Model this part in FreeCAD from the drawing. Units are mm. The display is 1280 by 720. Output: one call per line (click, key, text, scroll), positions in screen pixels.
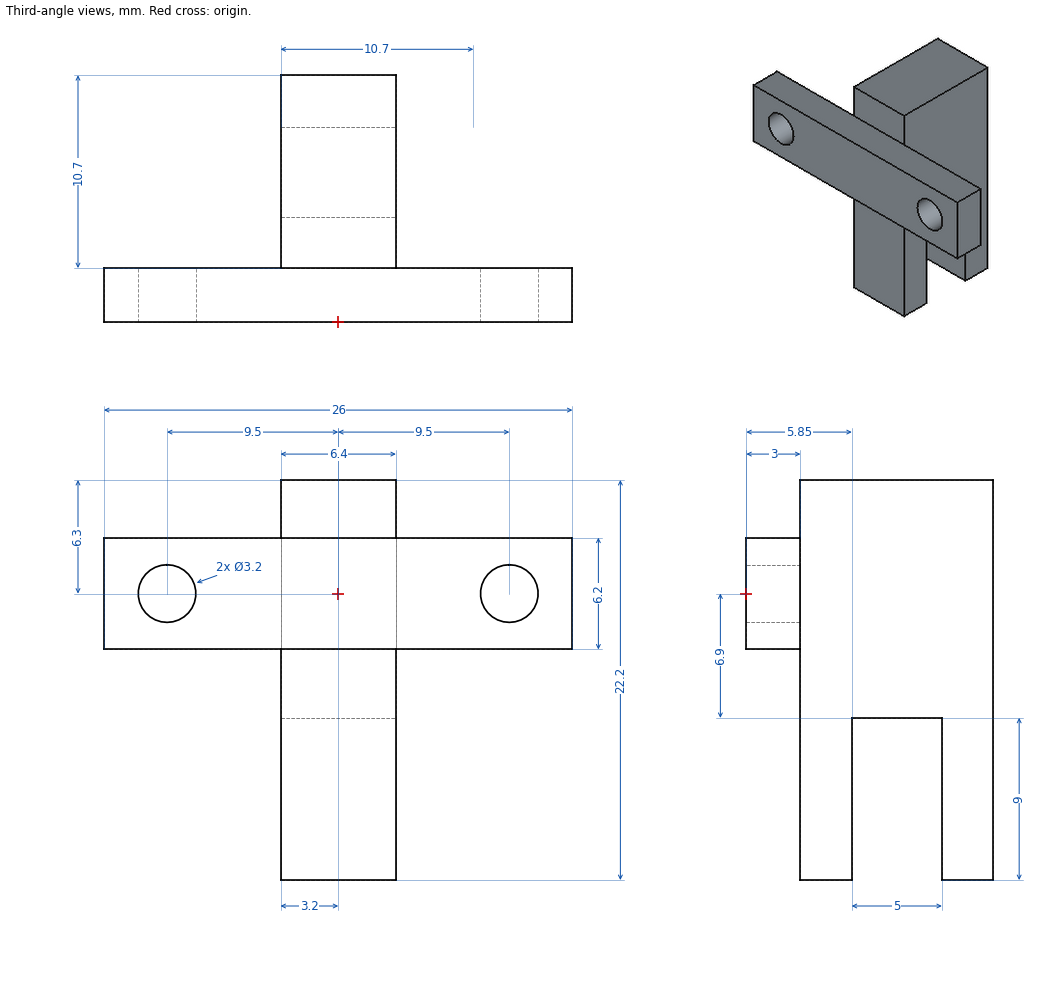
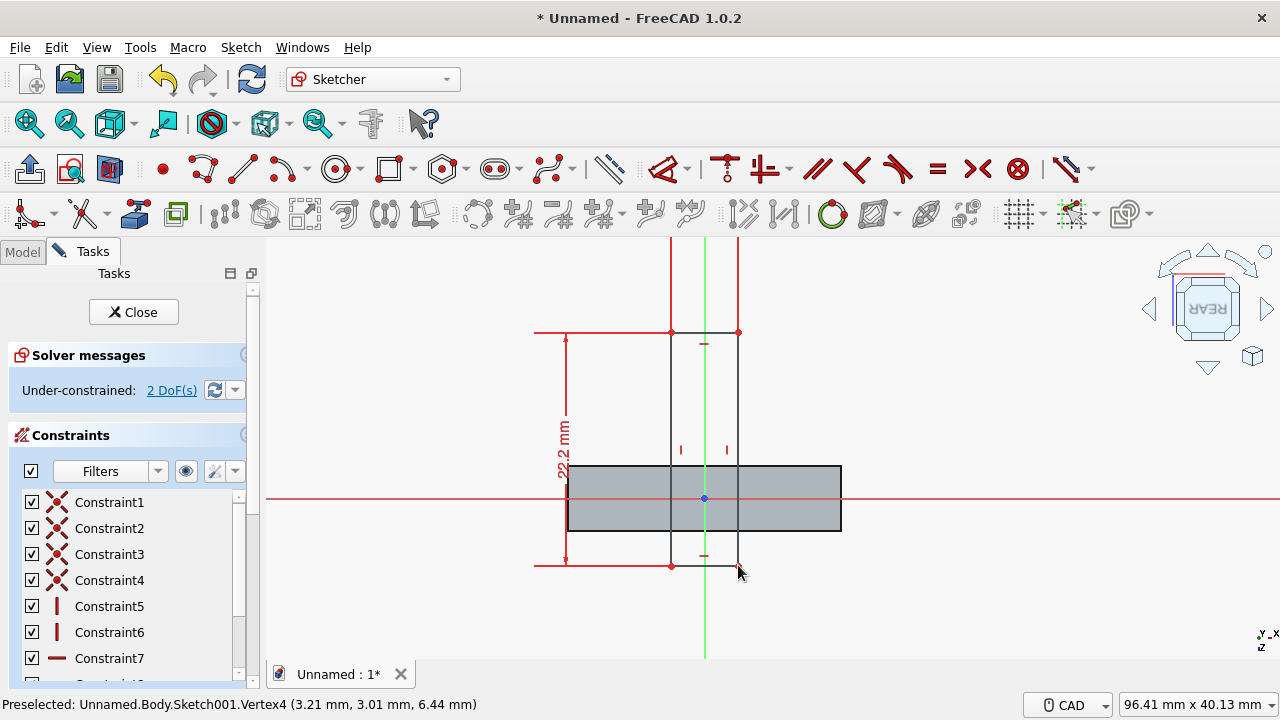
key(d)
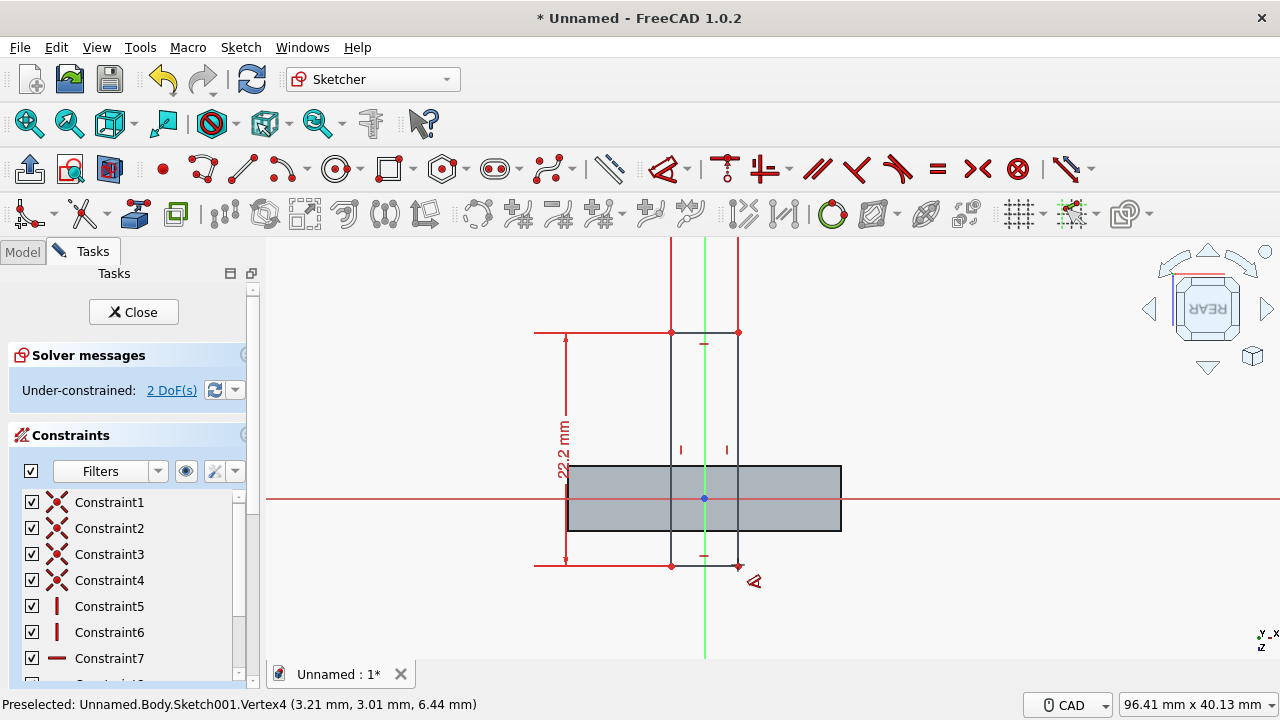
click(671, 333)
click(688, 299)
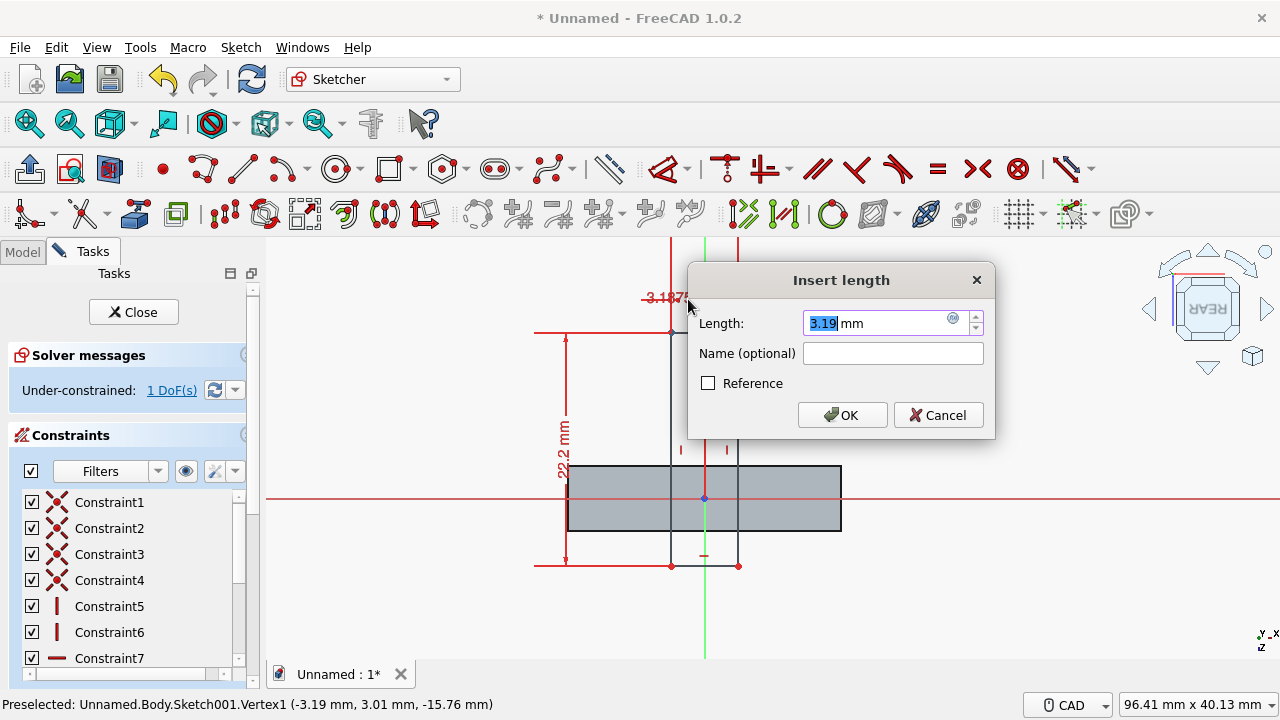
text(3.2)
key(Return)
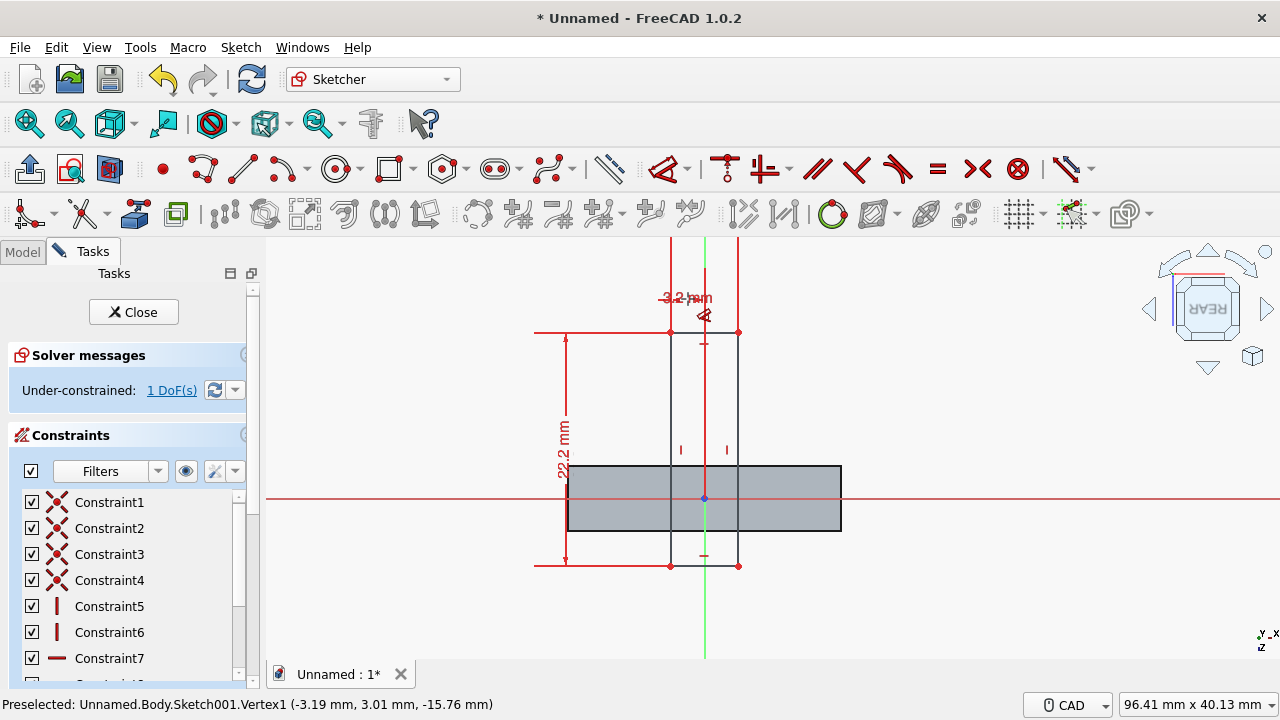
click(671, 566)
click(637, 533)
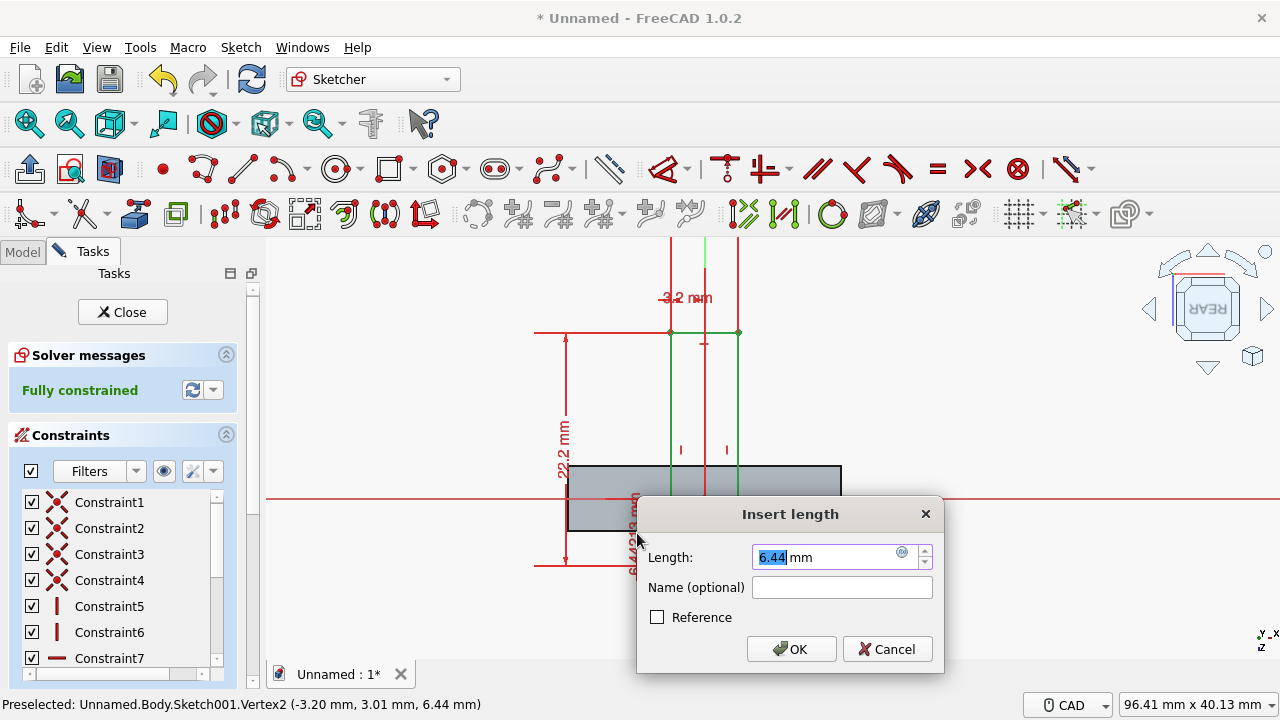
text(6.3)
key(Return)
key(Escape)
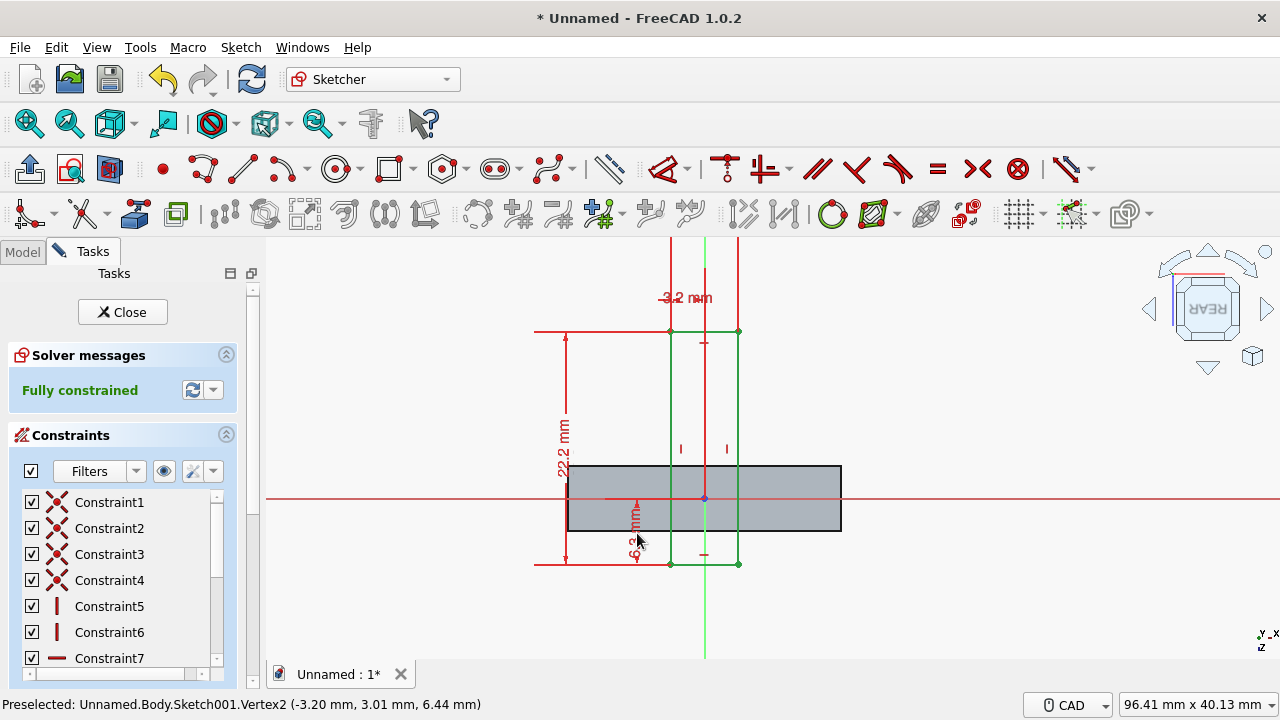
click(123, 312)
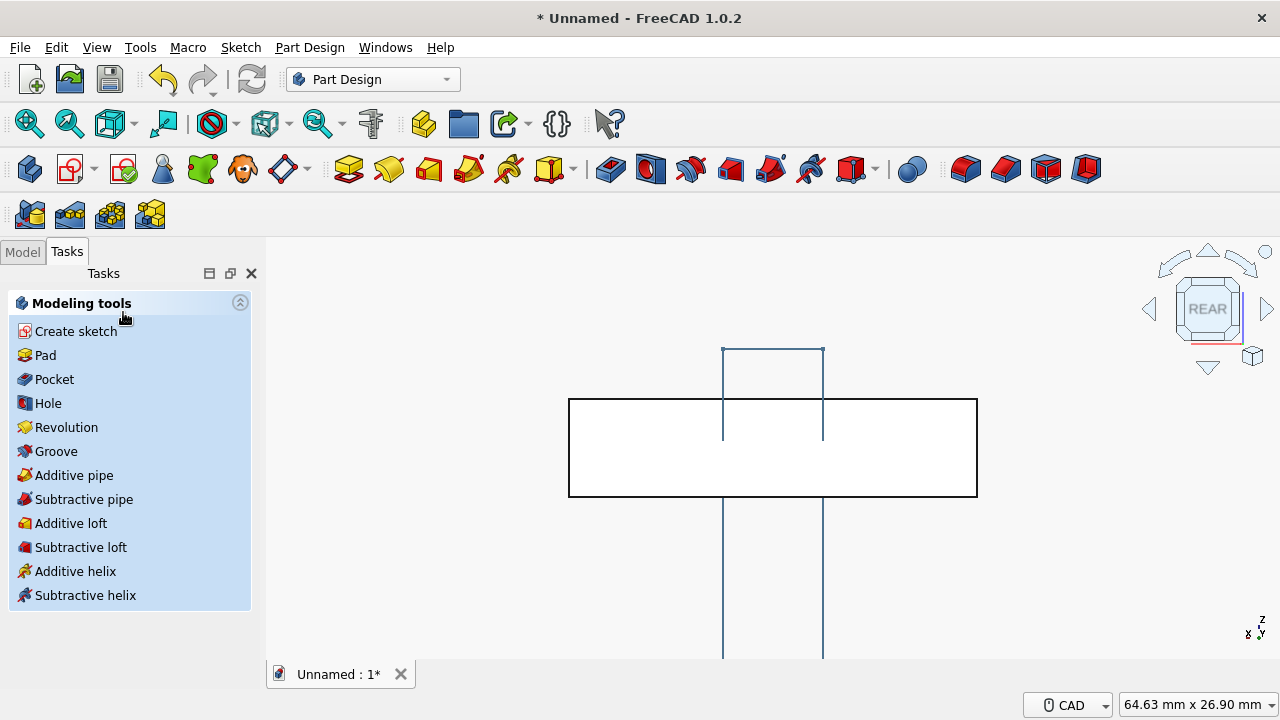
click(350, 170)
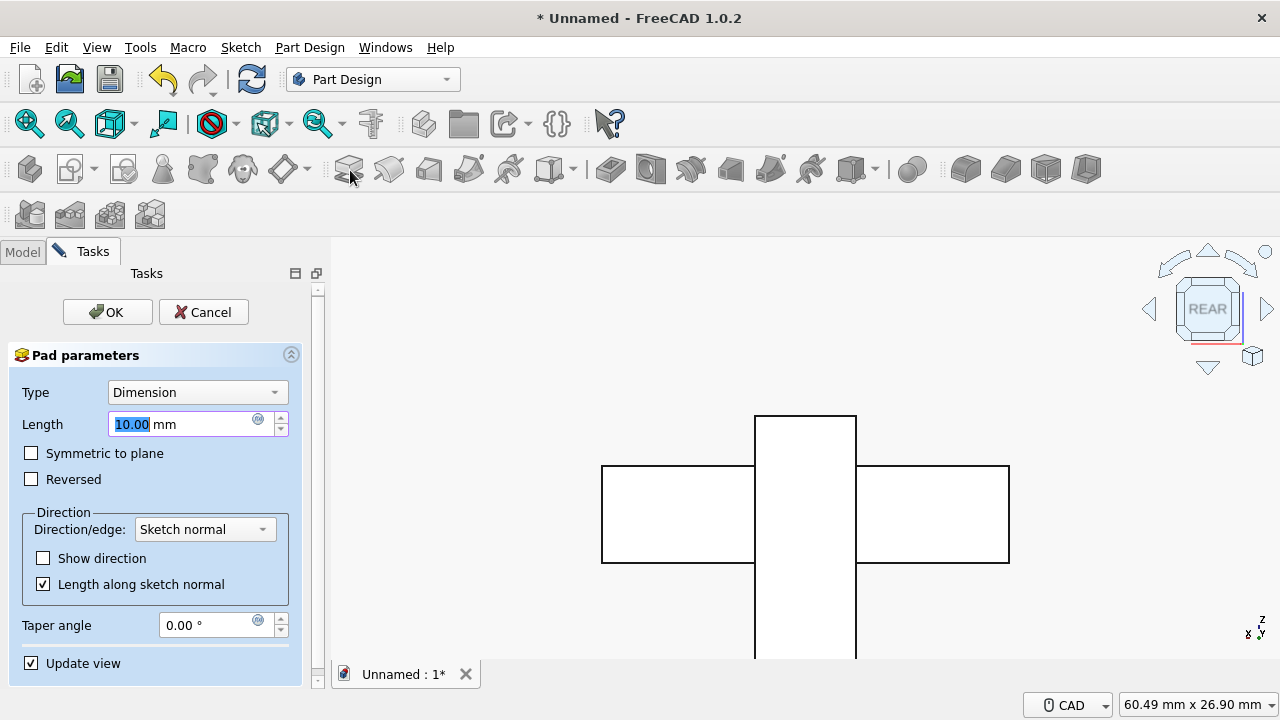
text(10.7)
key(Tab)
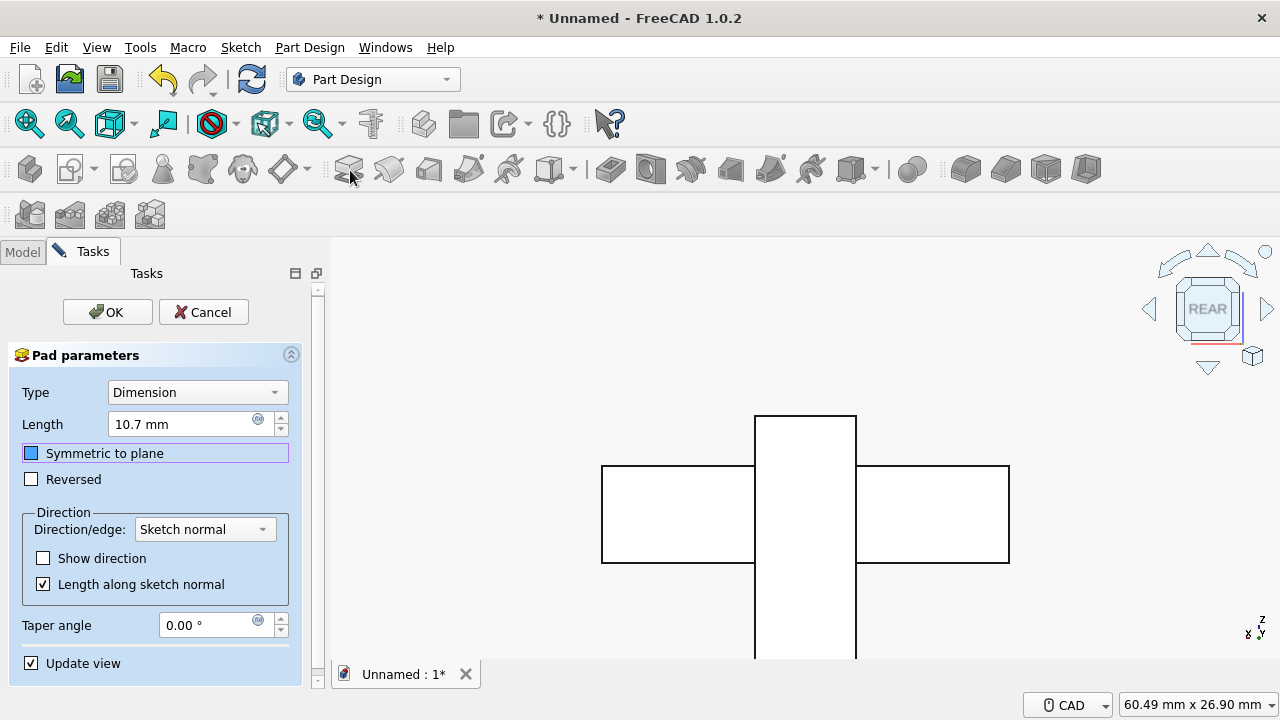
click(108, 312)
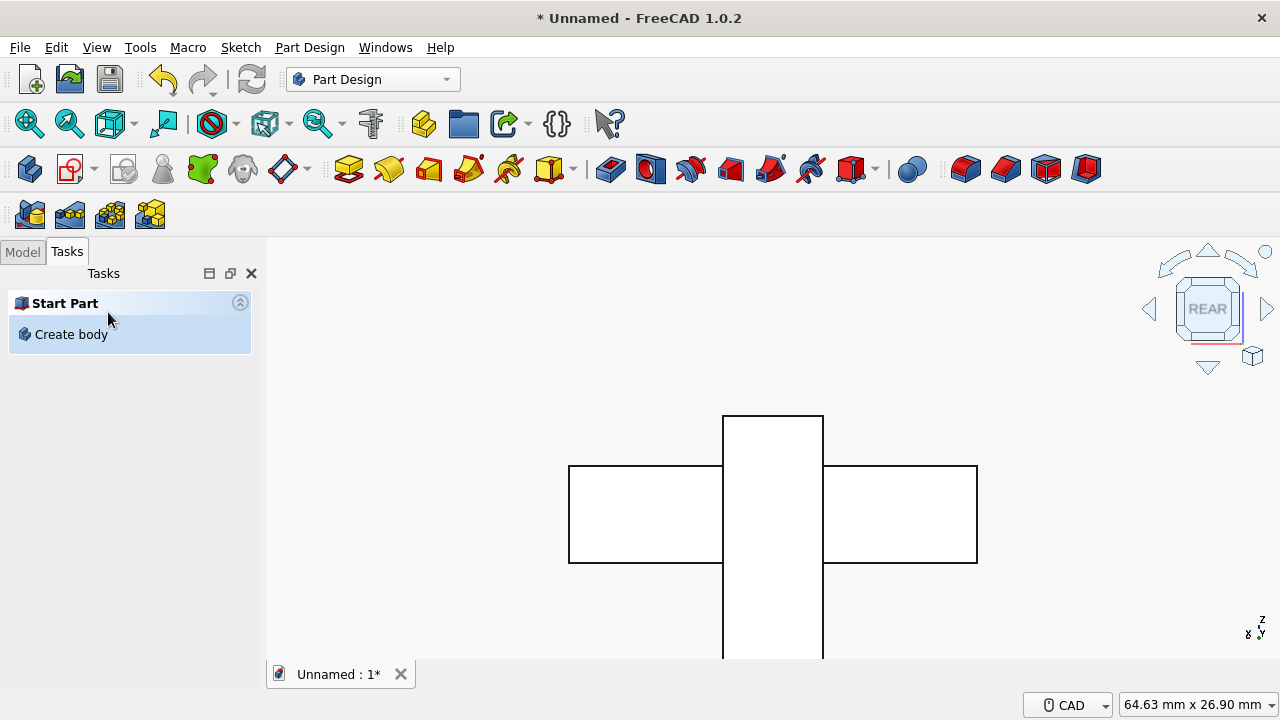
key(v)
key(f)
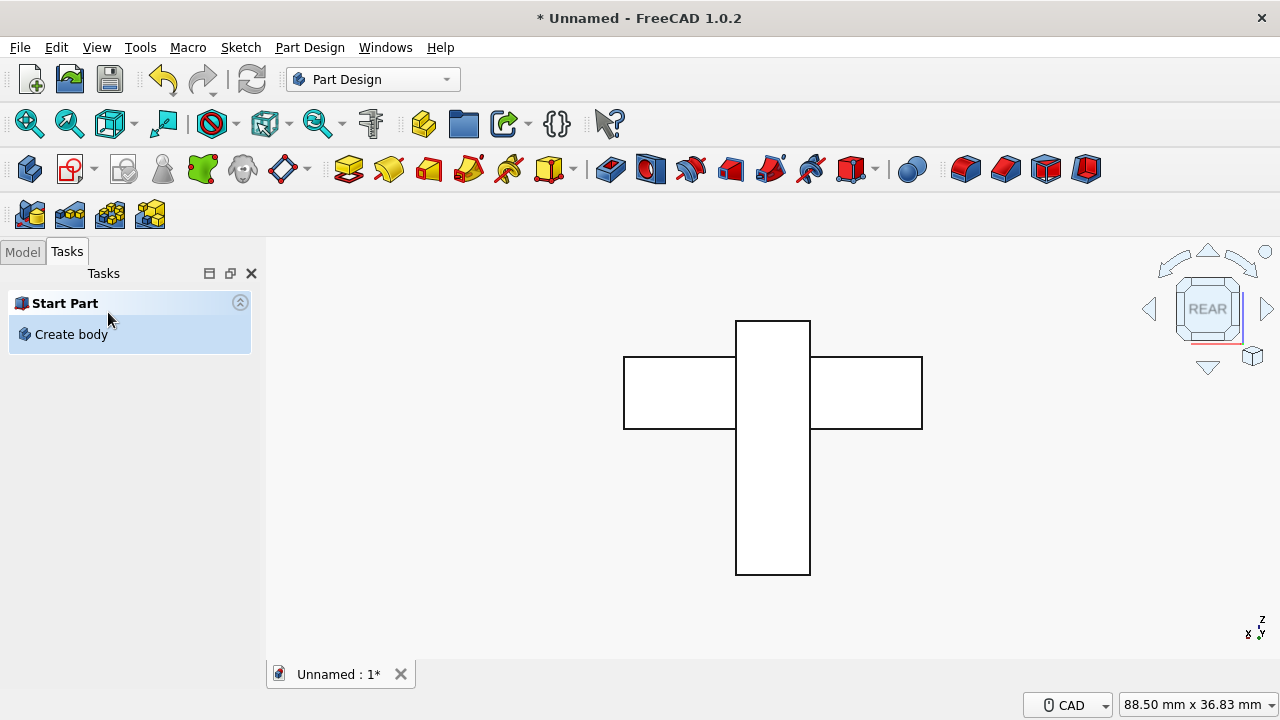
key(6)